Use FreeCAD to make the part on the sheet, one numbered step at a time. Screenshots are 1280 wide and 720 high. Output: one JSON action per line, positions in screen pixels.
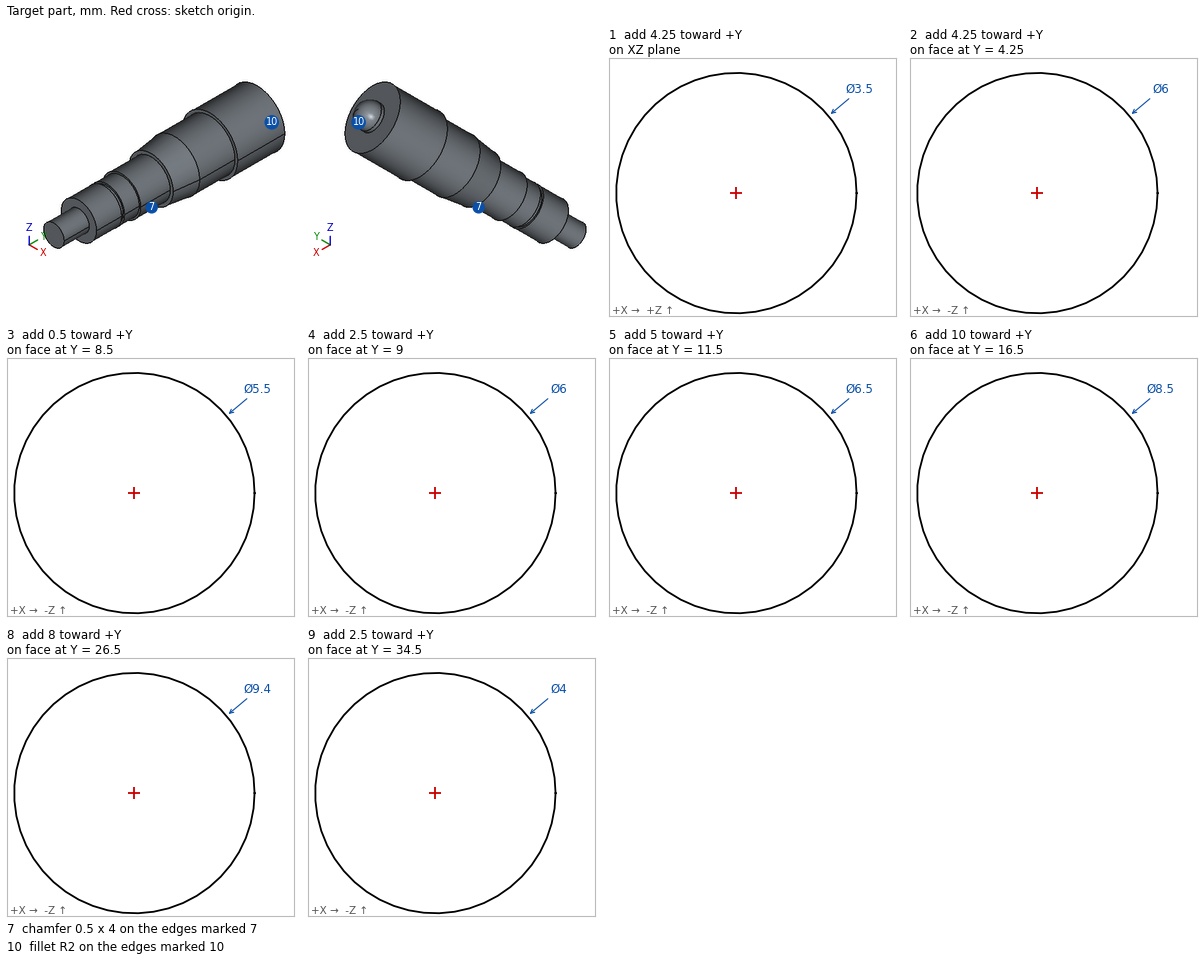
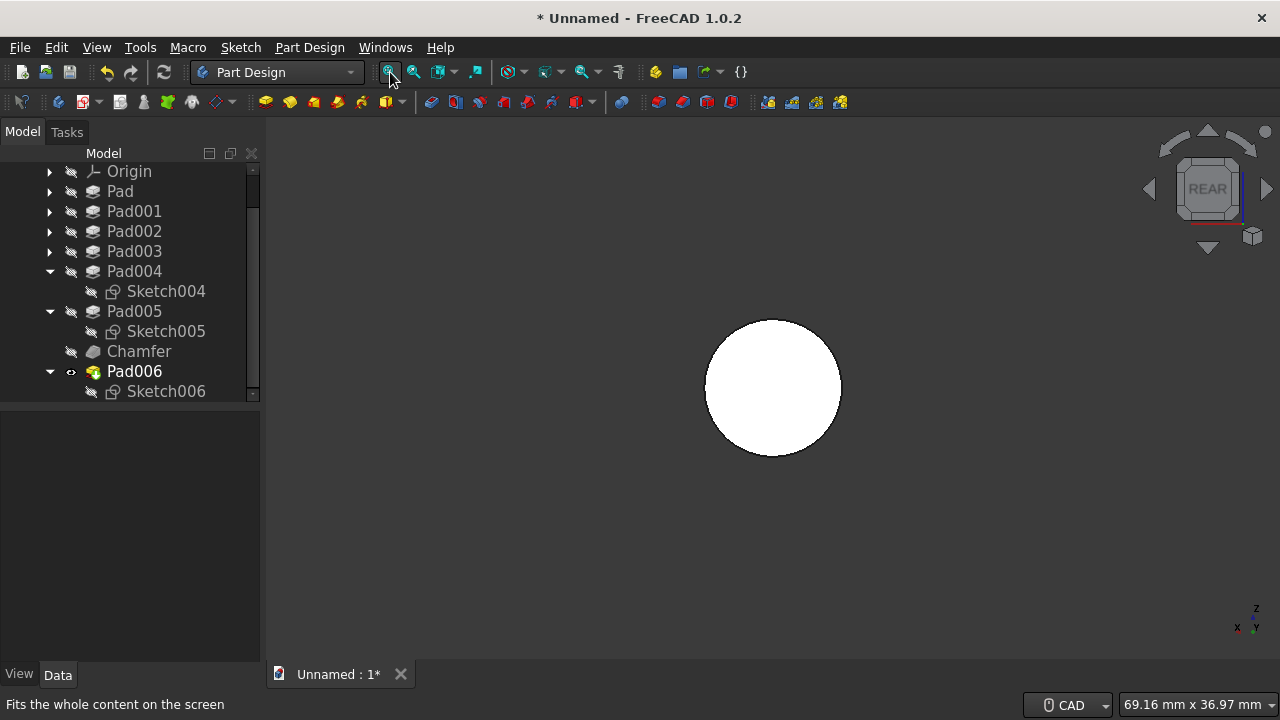
{"action": "left_click", "coordinate": [773, 387]}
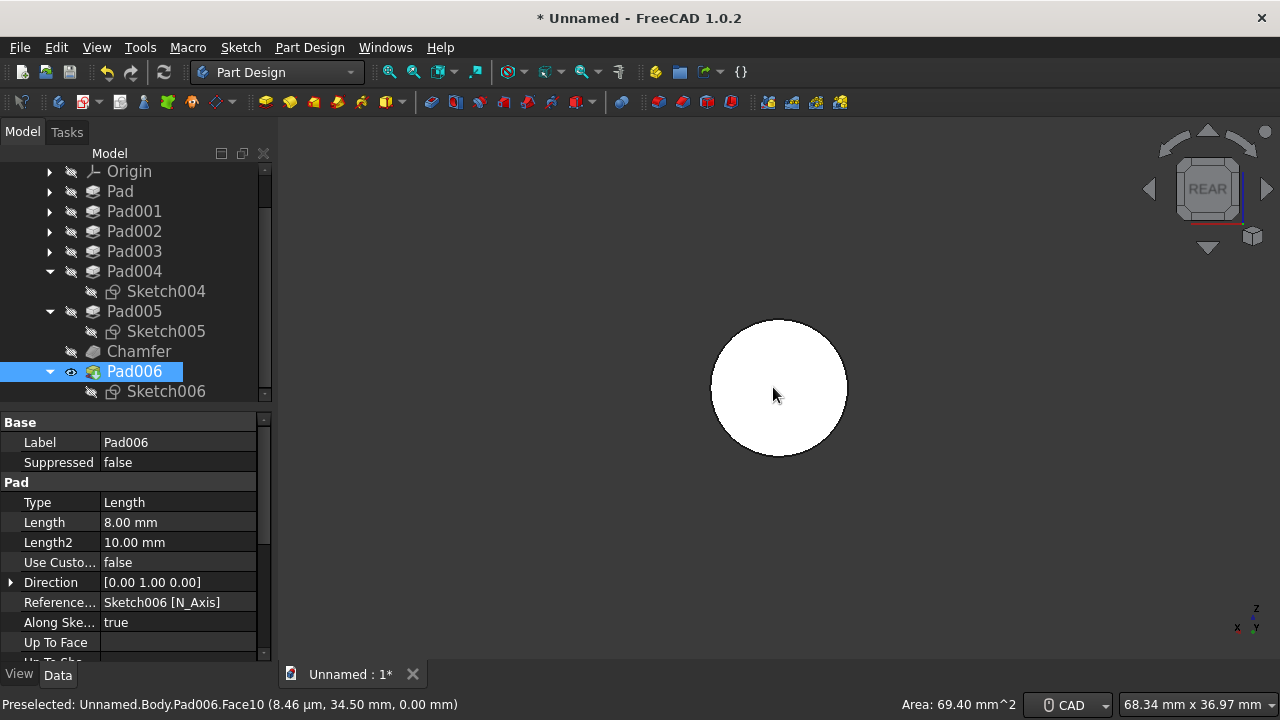
{"action": "left_click", "coordinate": [84, 102]}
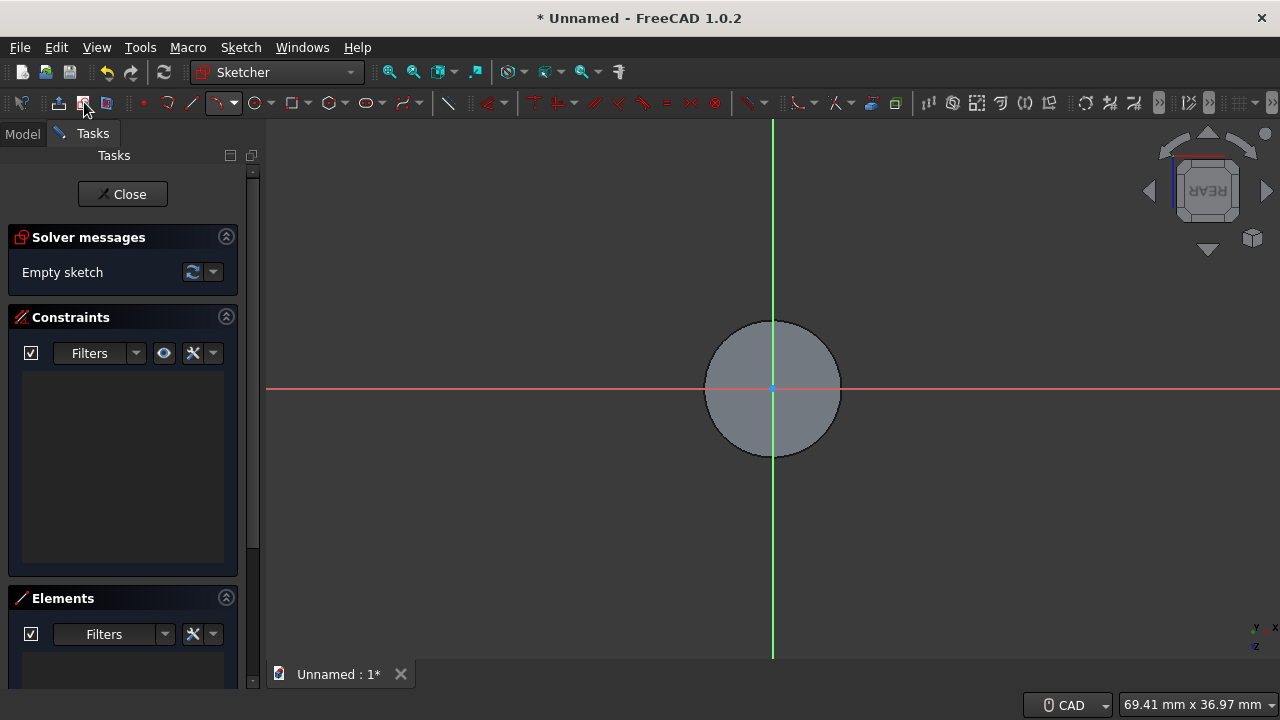
{"action": "scroll", "coordinate": [786, 389], "scroll_direction": "up", "scroll_amount": 9}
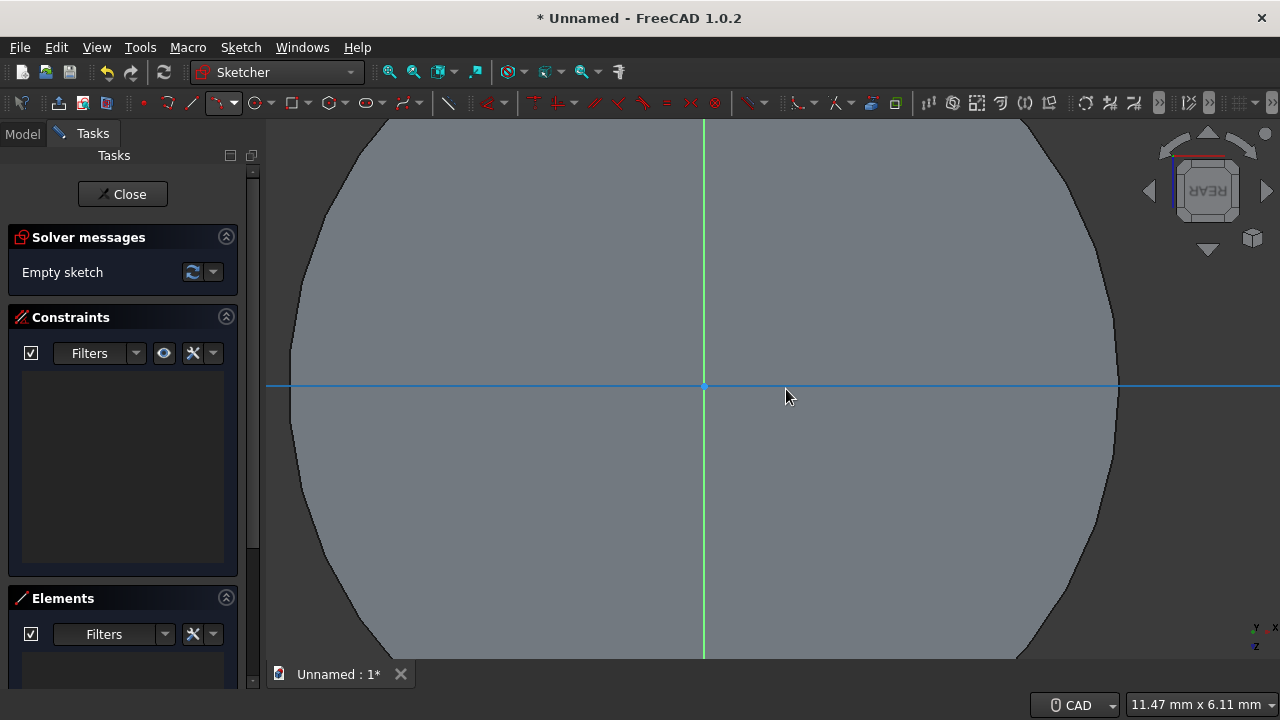
{"action": "left_click", "coordinate": [256, 104]}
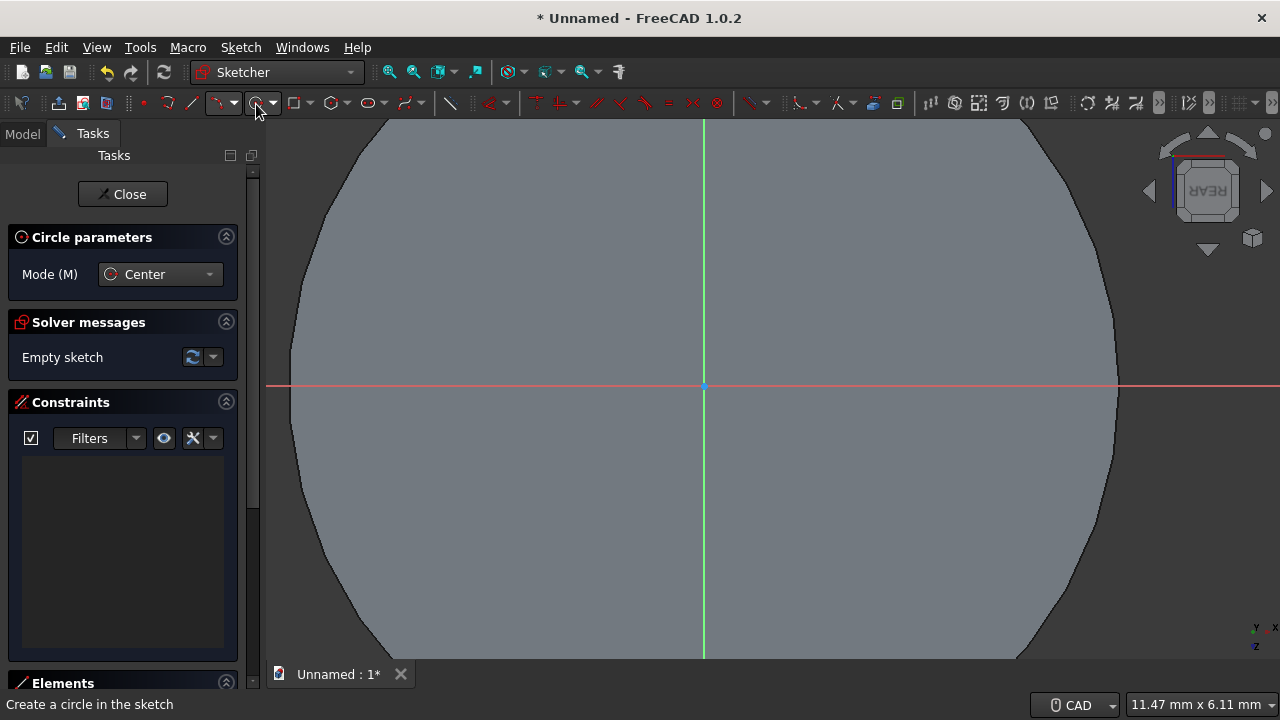
{"action": "left_click", "coordinate": [704, 386]}
{"action": "mouse_move", "coordinate": [829, 261]}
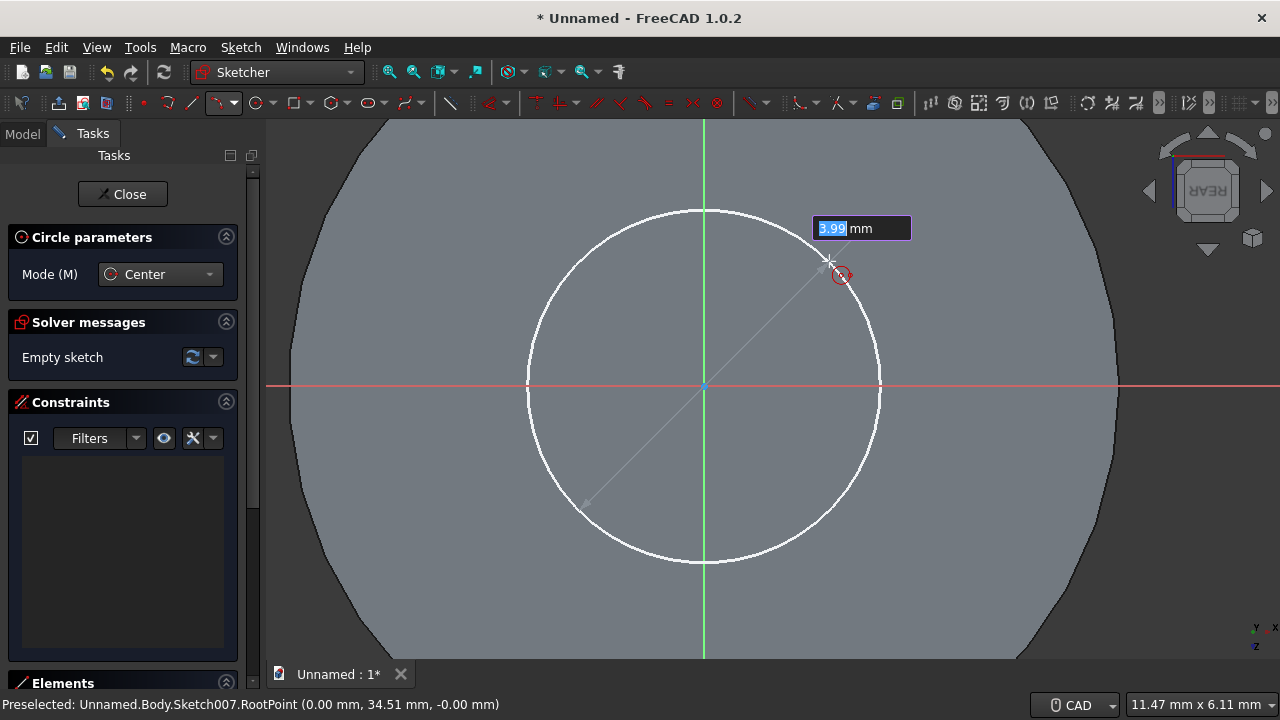
{"action": "type", "text": "4"}
{"action": "key", "text": "Return"}
{"action": "key", "text": "Escape"}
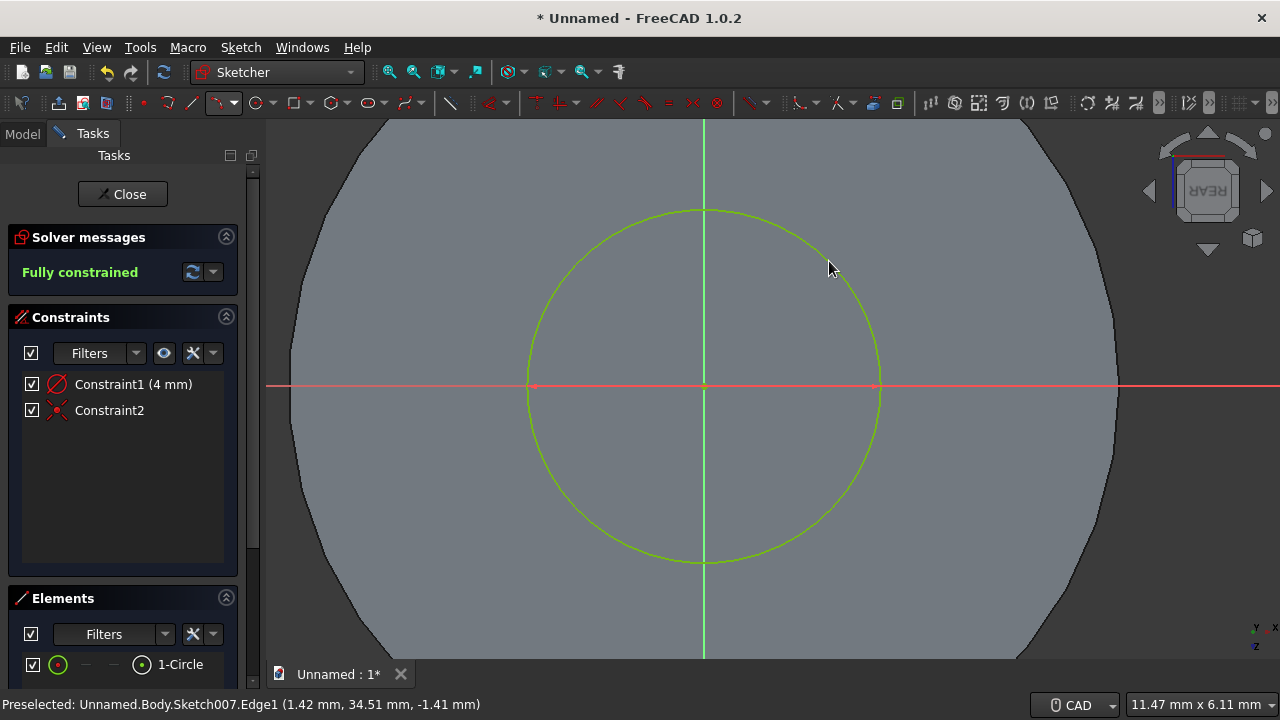
{"action": "left_click", "coordinate": [123, 194]}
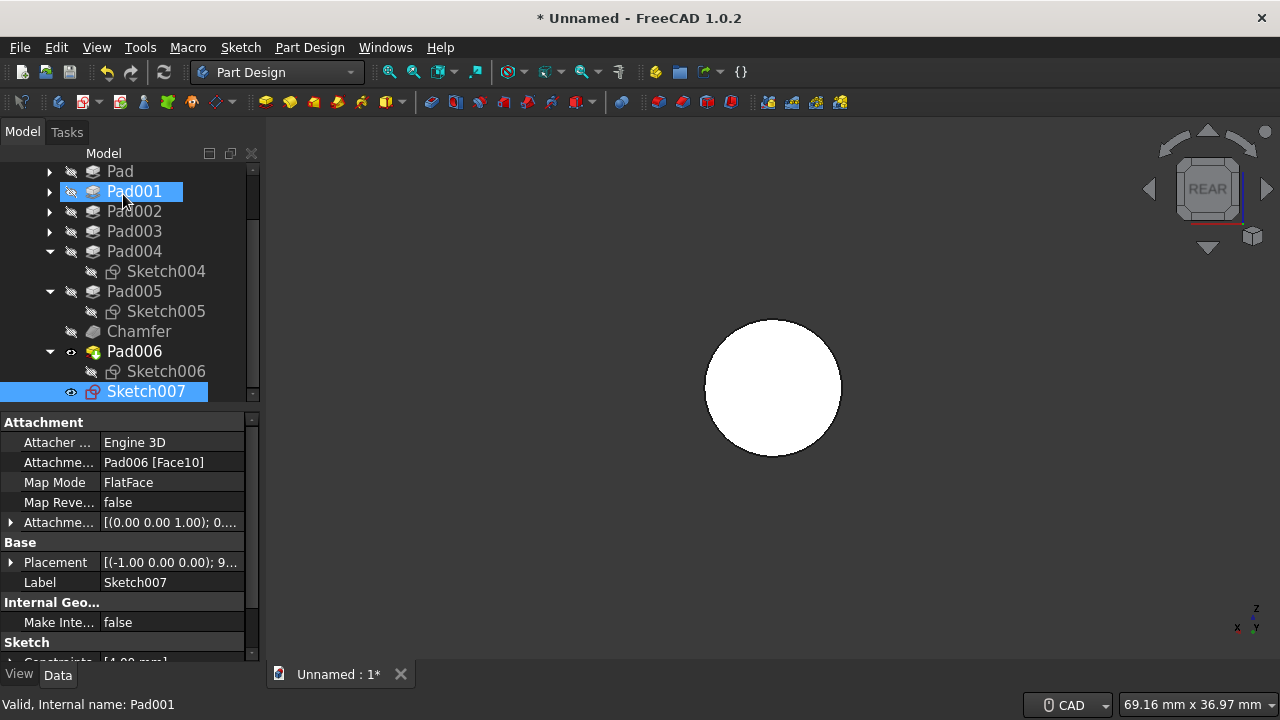
{"action": "left_click", "coordinate": [266, 102]}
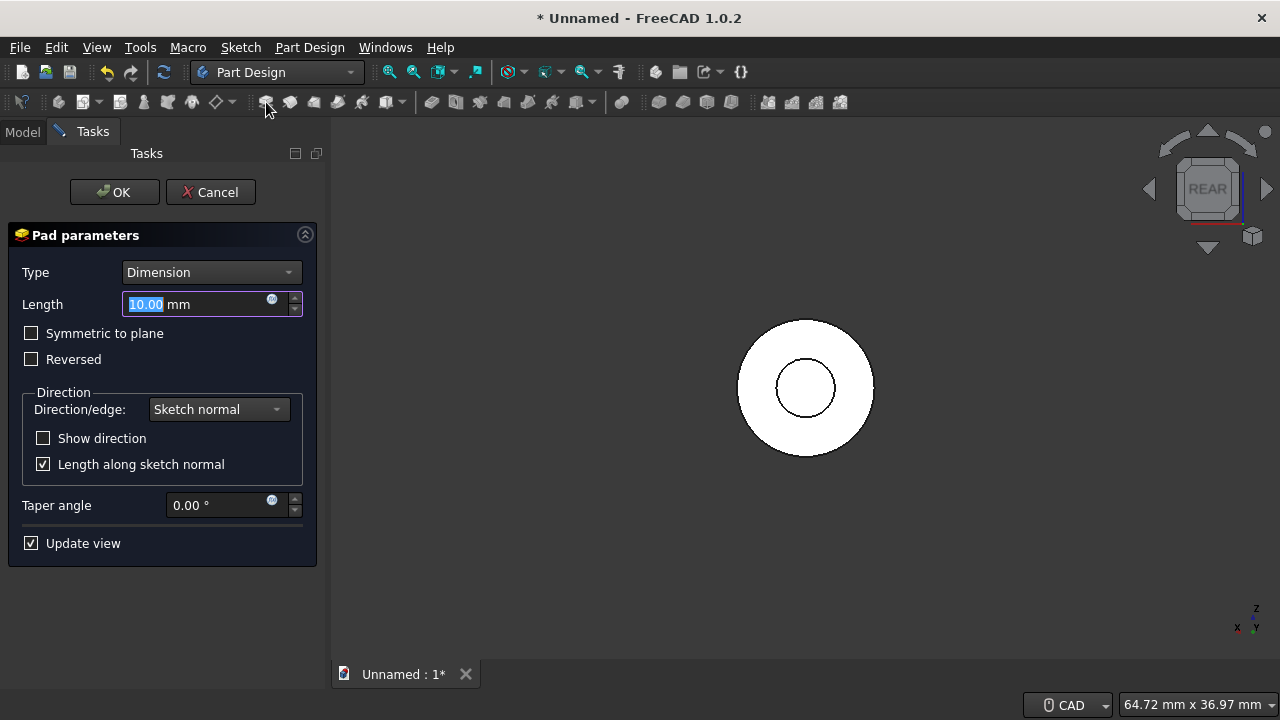
{"action": "type", "text": "2.5"}
{"action": "key", "text": "Tab"}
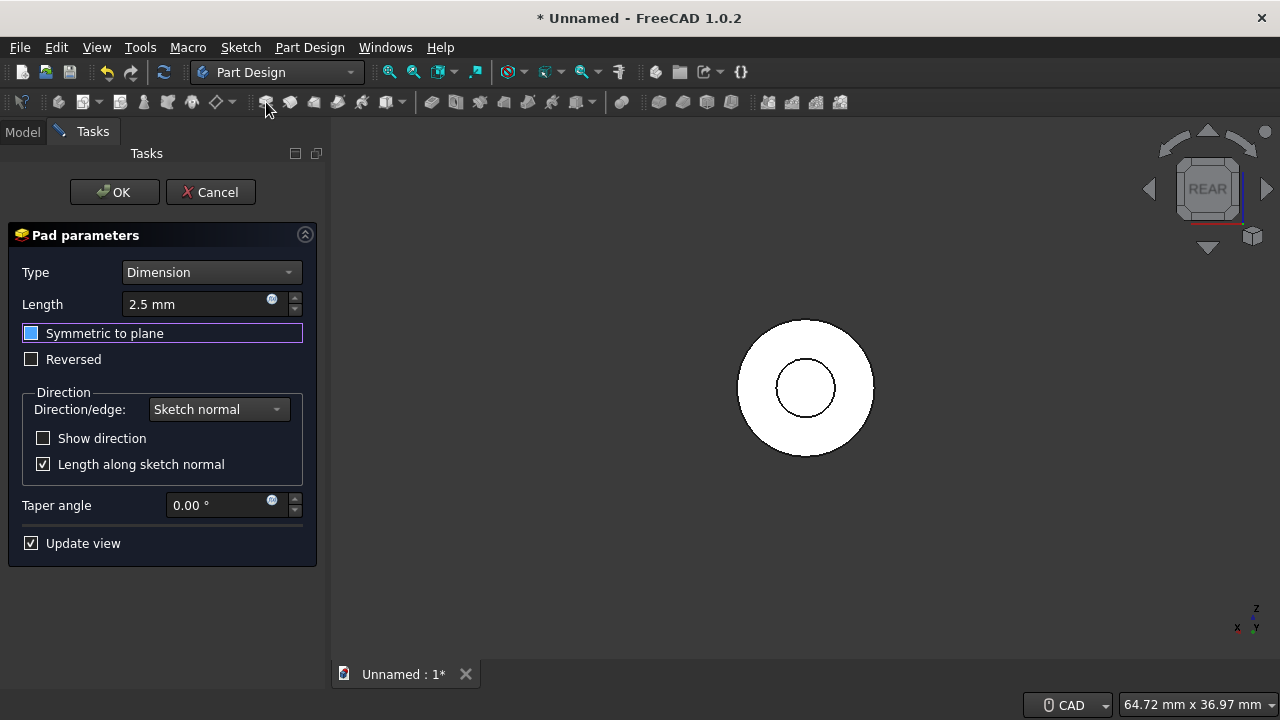
{"action": "left_click", "coordinate": [115, 192]}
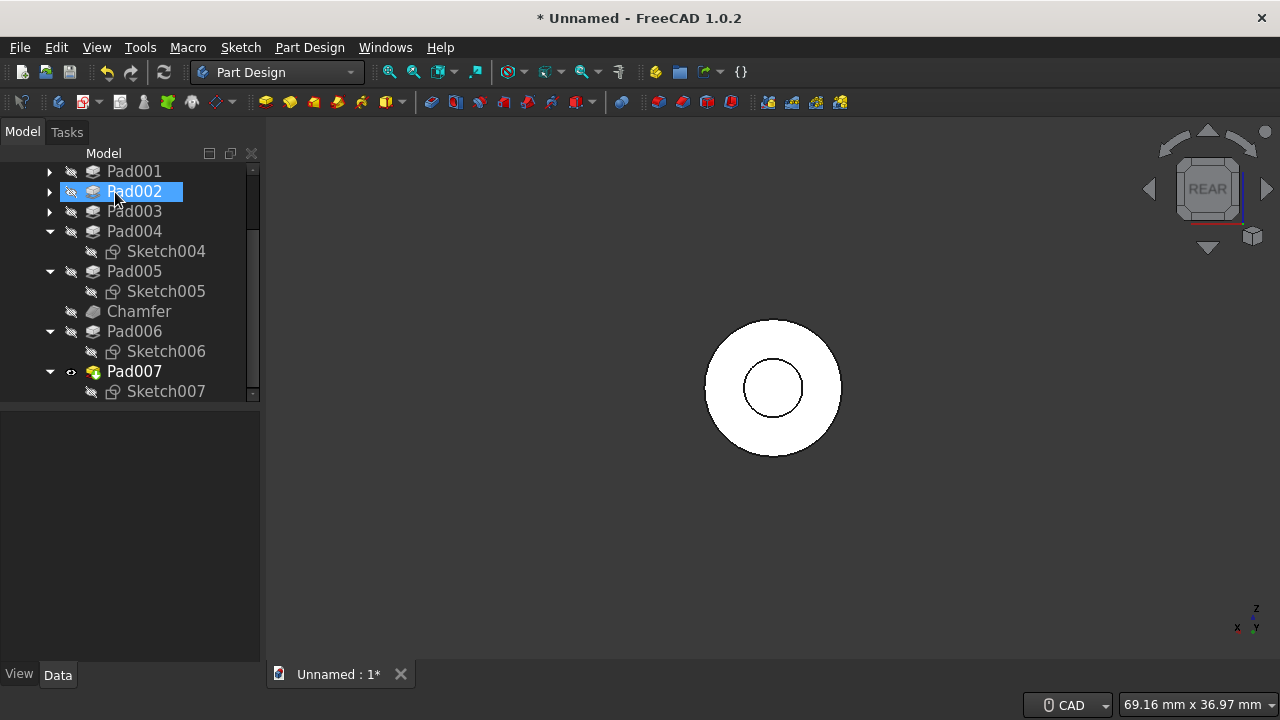
{"action": "key", "text": "v f"}